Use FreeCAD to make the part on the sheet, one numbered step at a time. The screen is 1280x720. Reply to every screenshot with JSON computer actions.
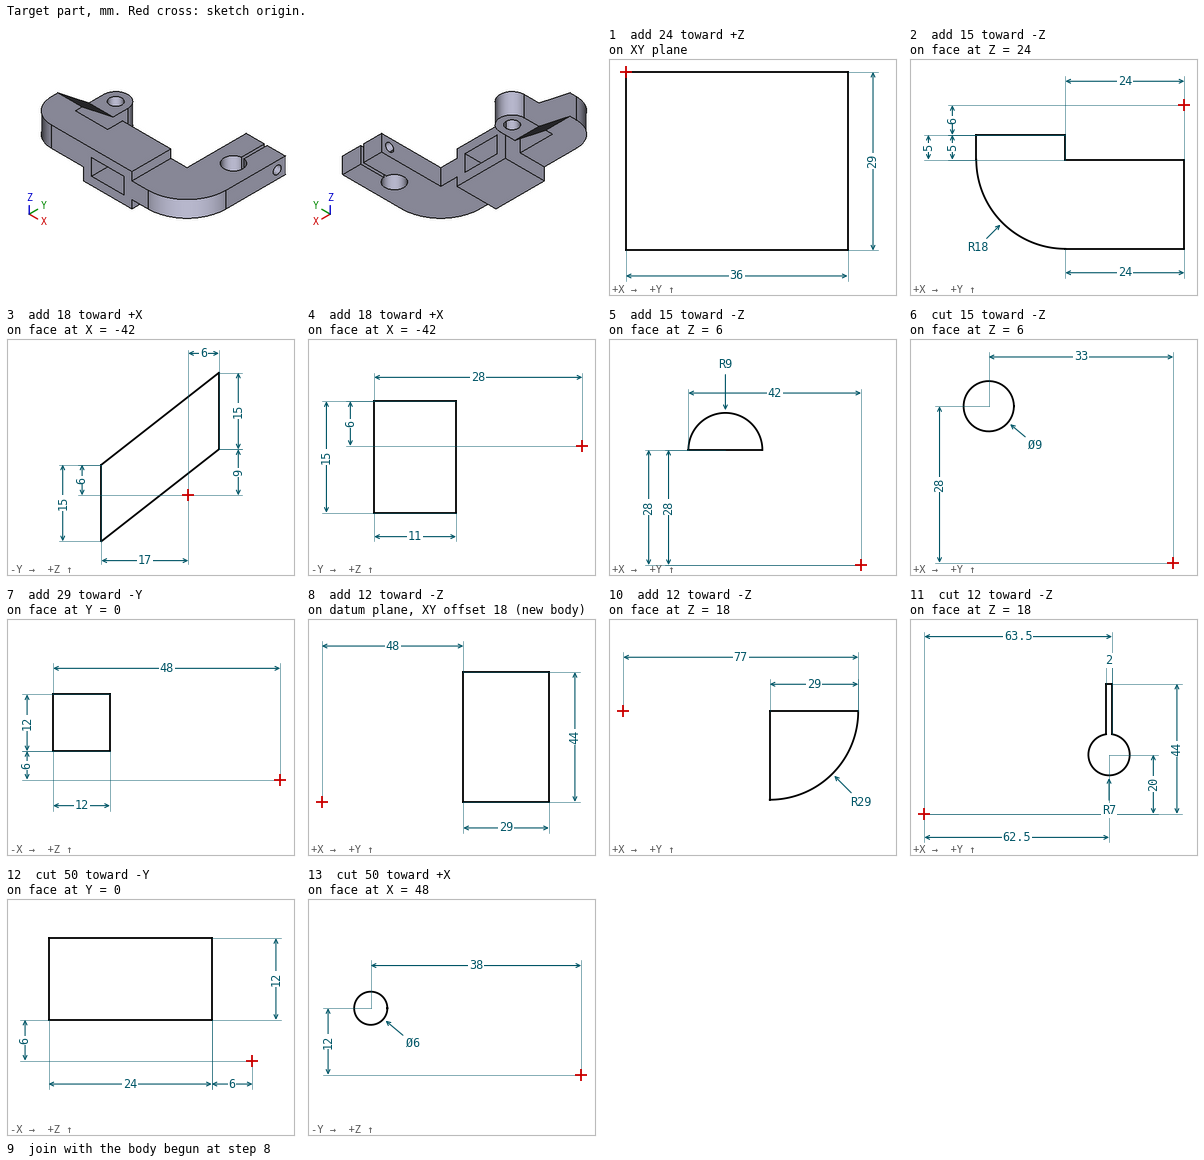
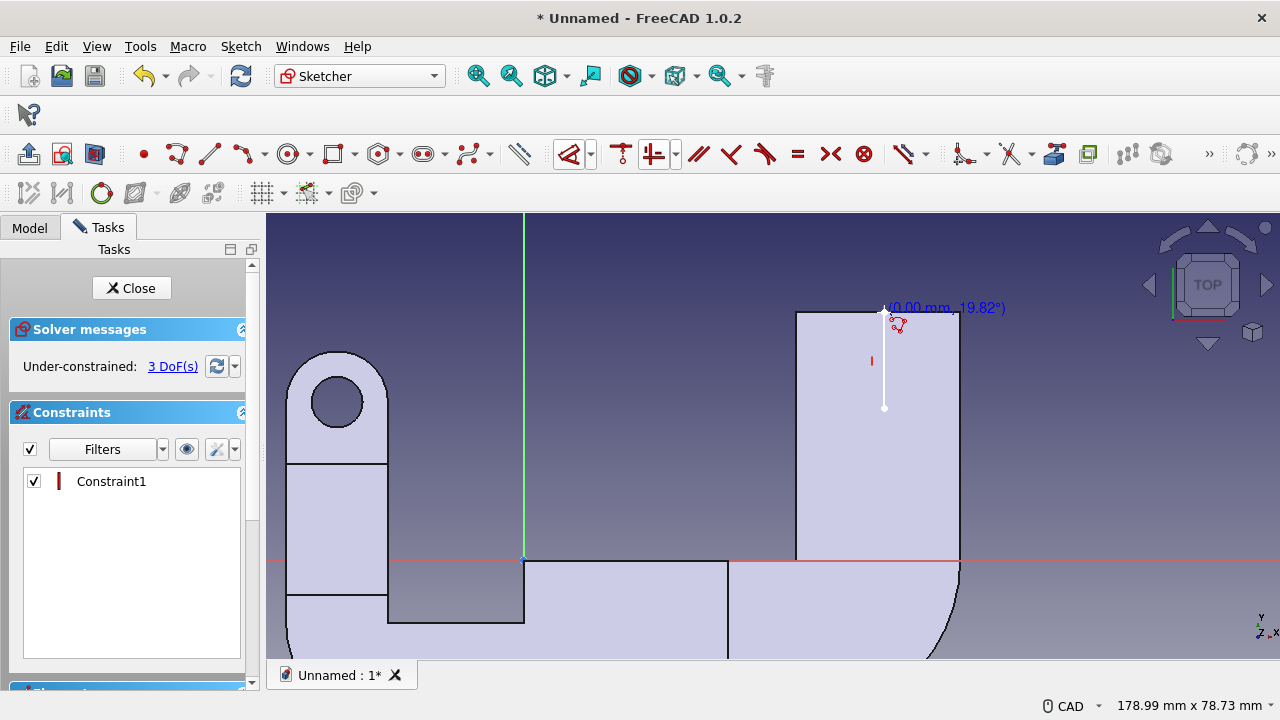
{"action": "scroll", "coordinate": [872, 312], "scroll_direction": "up", "scroll_amount": 2}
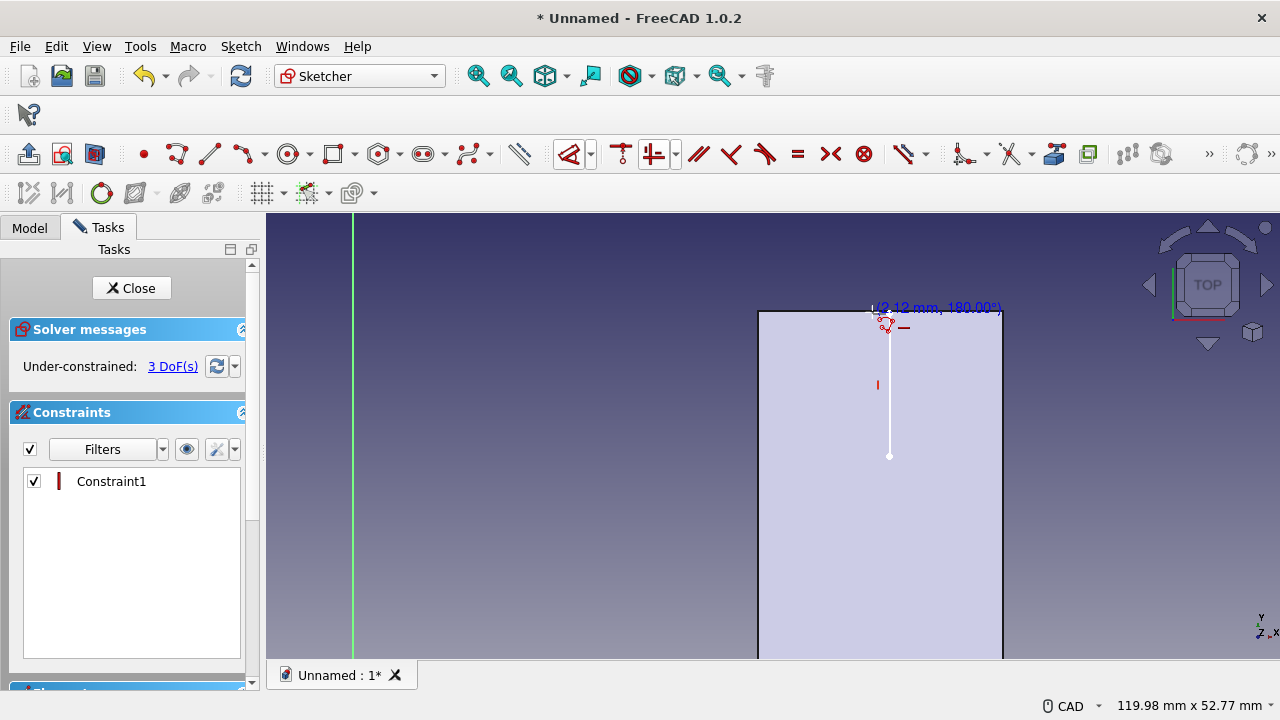
{"action": "left_click", "coordinate": [872, 312]}
{"action": "left_click", "coordinate": [872, 455]}
{"action": "right_click", "coordinate": [872, 455]}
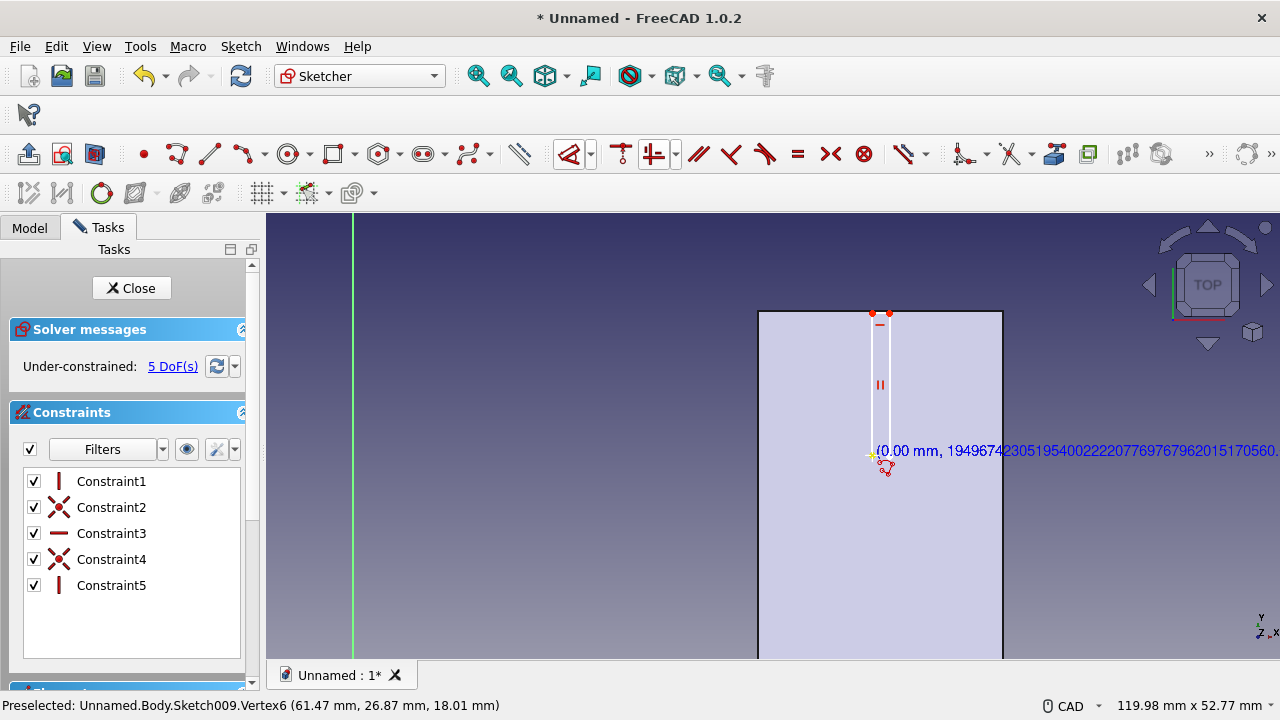
{"action": "left_click", "coordinate": [242, 154]}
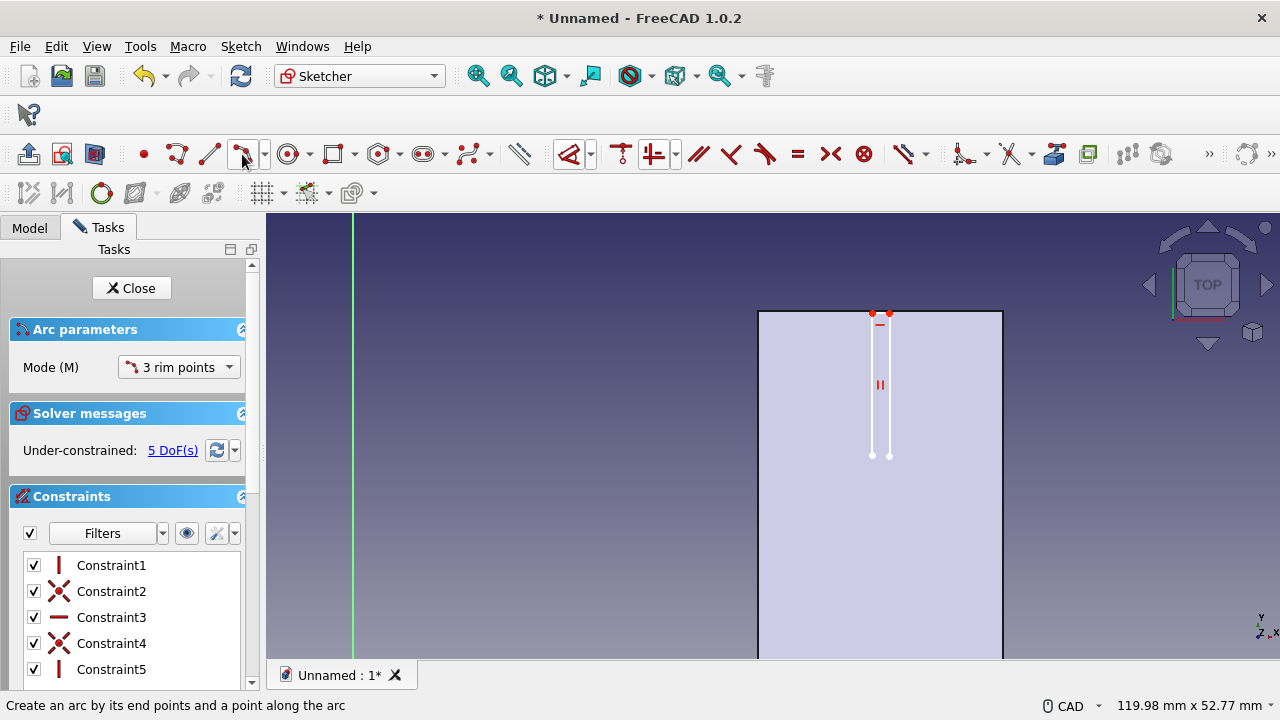
{"action": "left_click", "coordinate": [872, 456]}
{"action": "left_click", "coordinate": [890, 457]}
{"action": "left_click", "coordinate": [881, 573]}
{"action": "key", "text": "Escape"}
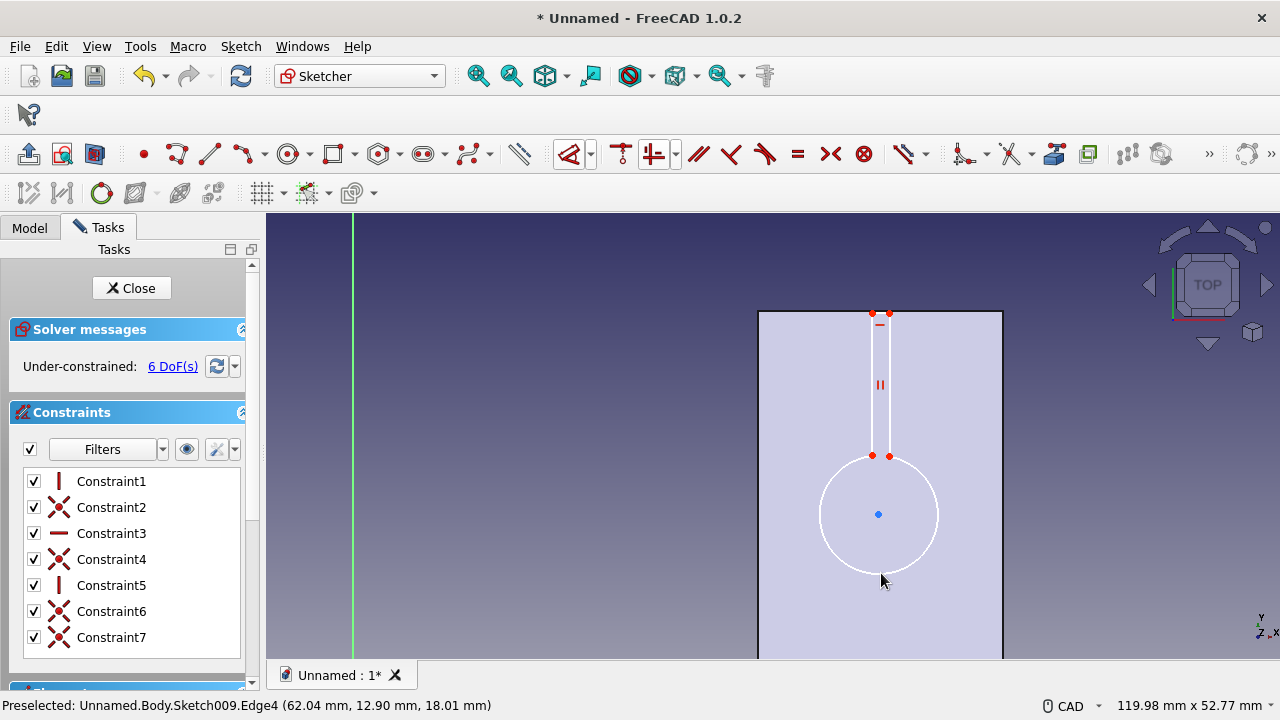
{"action": "left_click", "coordinate": [823, 535]}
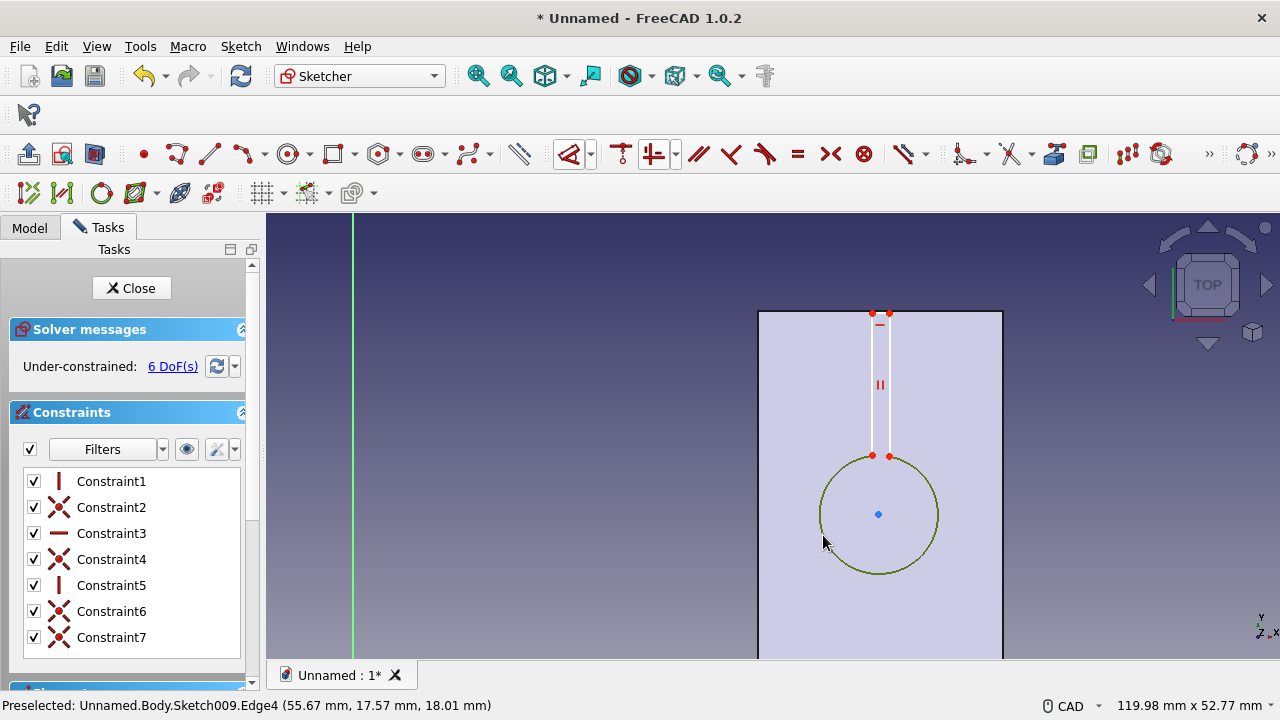
{"action": "key", "text": "k r"}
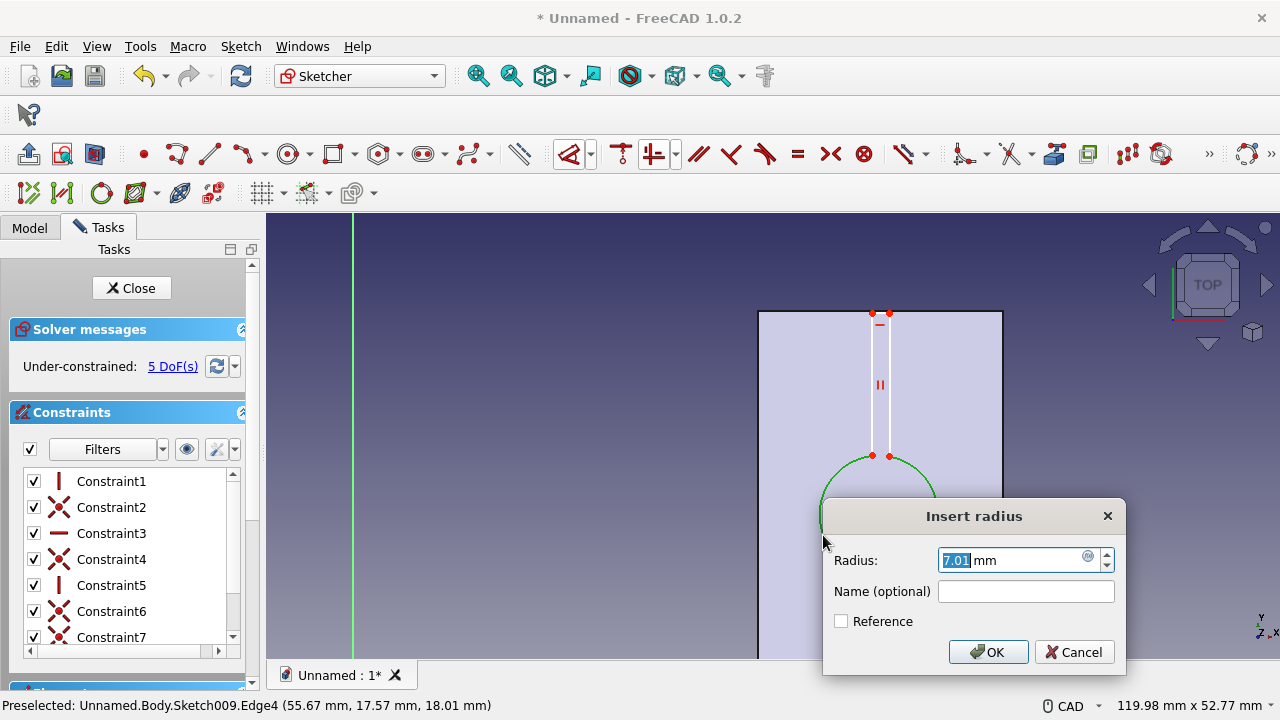
{"action": "type", "text": "7"}
{"action": "key", "text": "Return"}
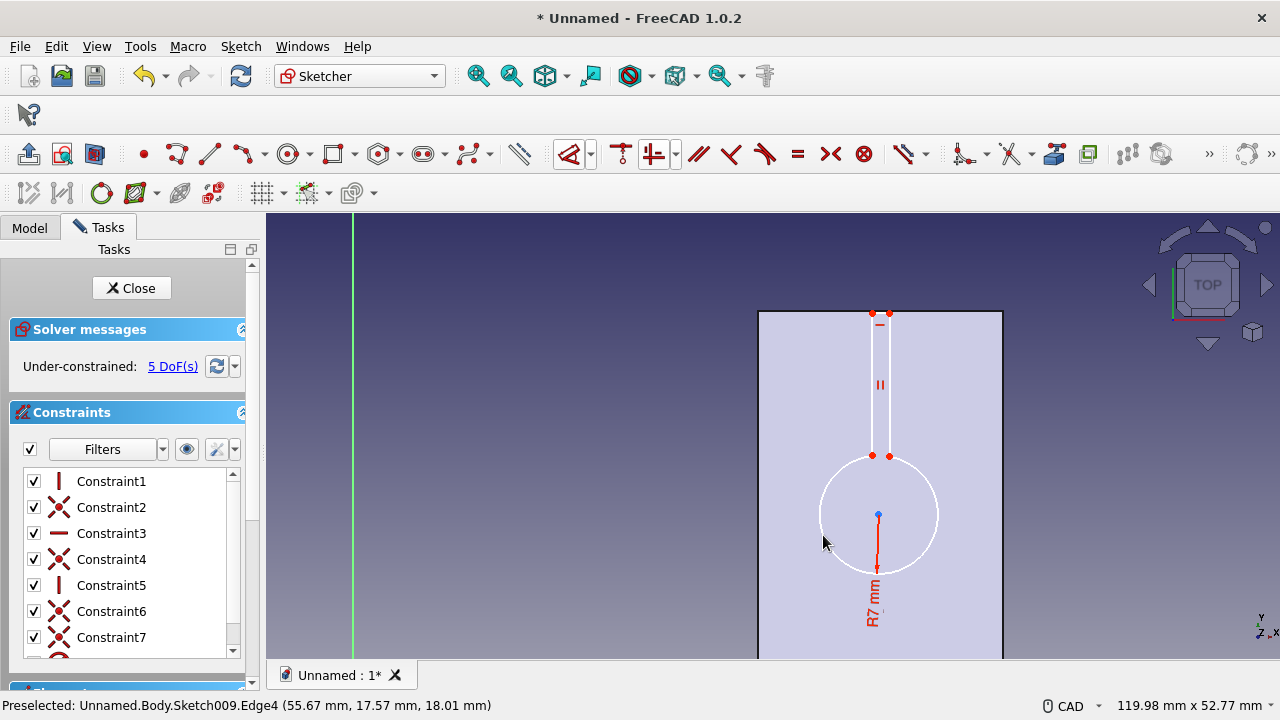
{"action": "scroll", "coordinate": [881, 313], "scroll_direction": "up", "scroll_amount": 5}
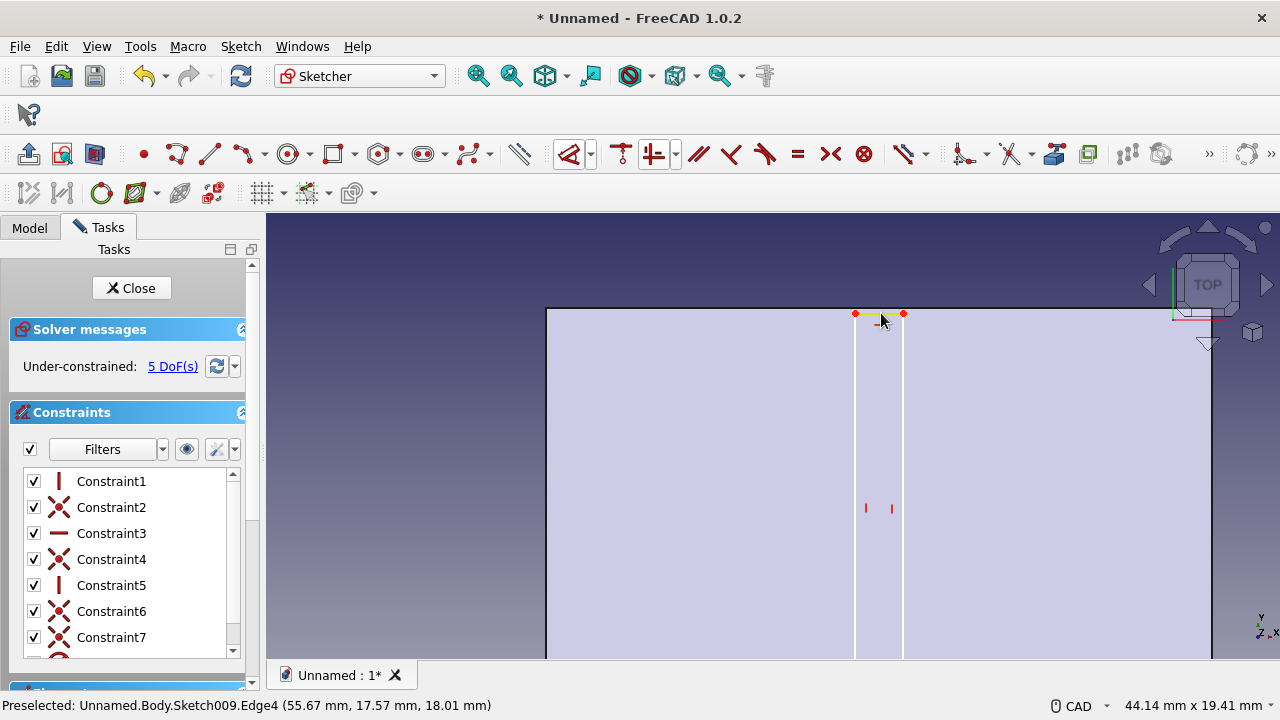
{"action": "left_click", "coordinate": [879, 314]}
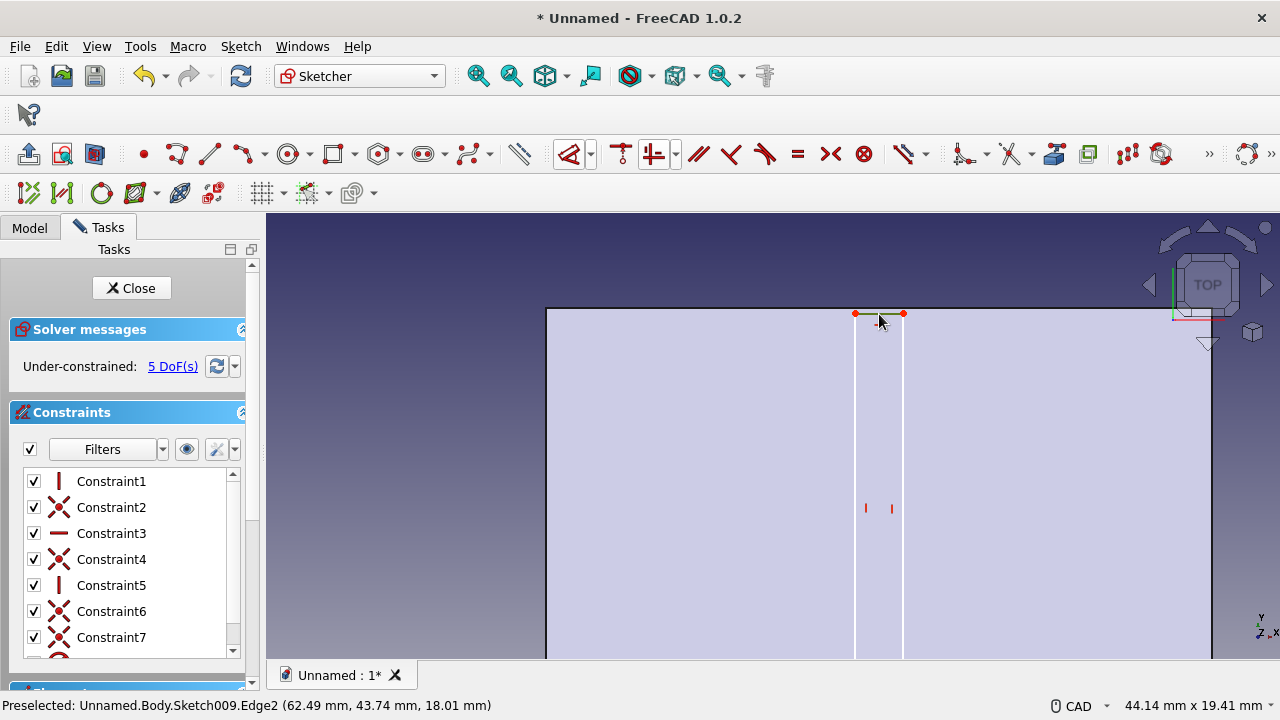
{"action": "left_click", "coordinate": [590, 154]}